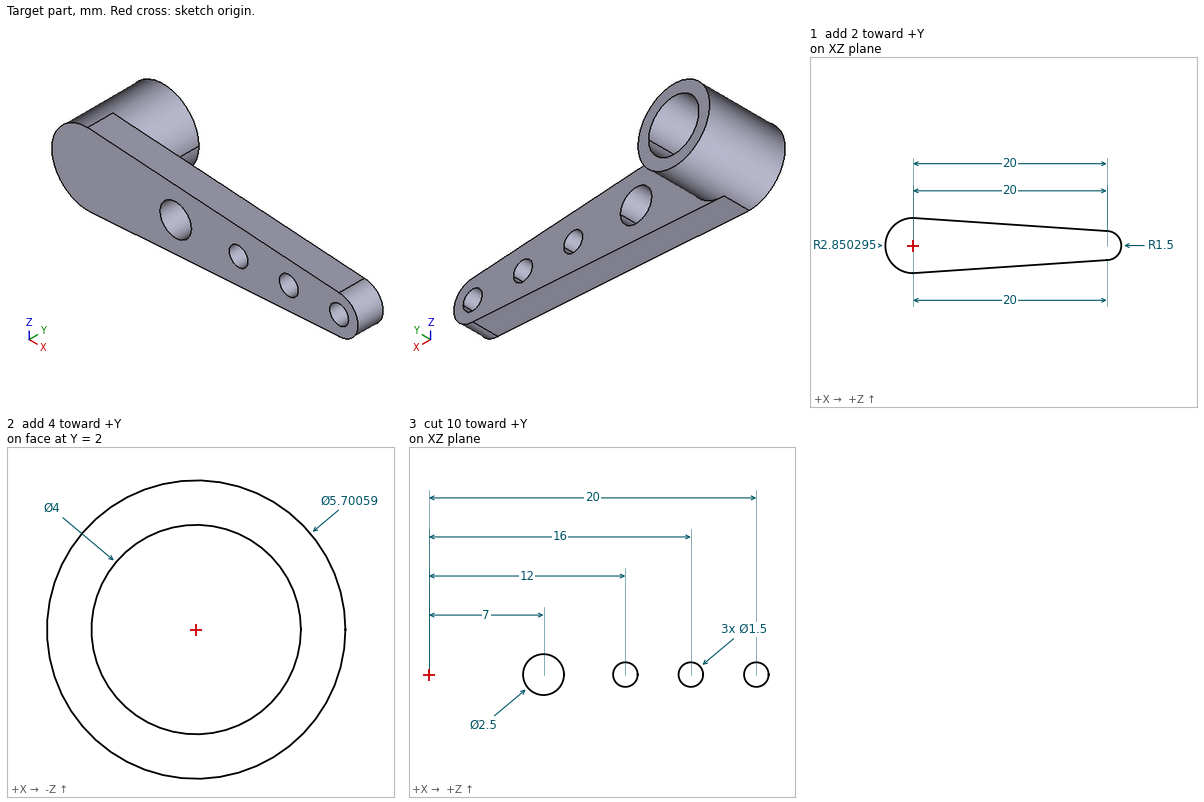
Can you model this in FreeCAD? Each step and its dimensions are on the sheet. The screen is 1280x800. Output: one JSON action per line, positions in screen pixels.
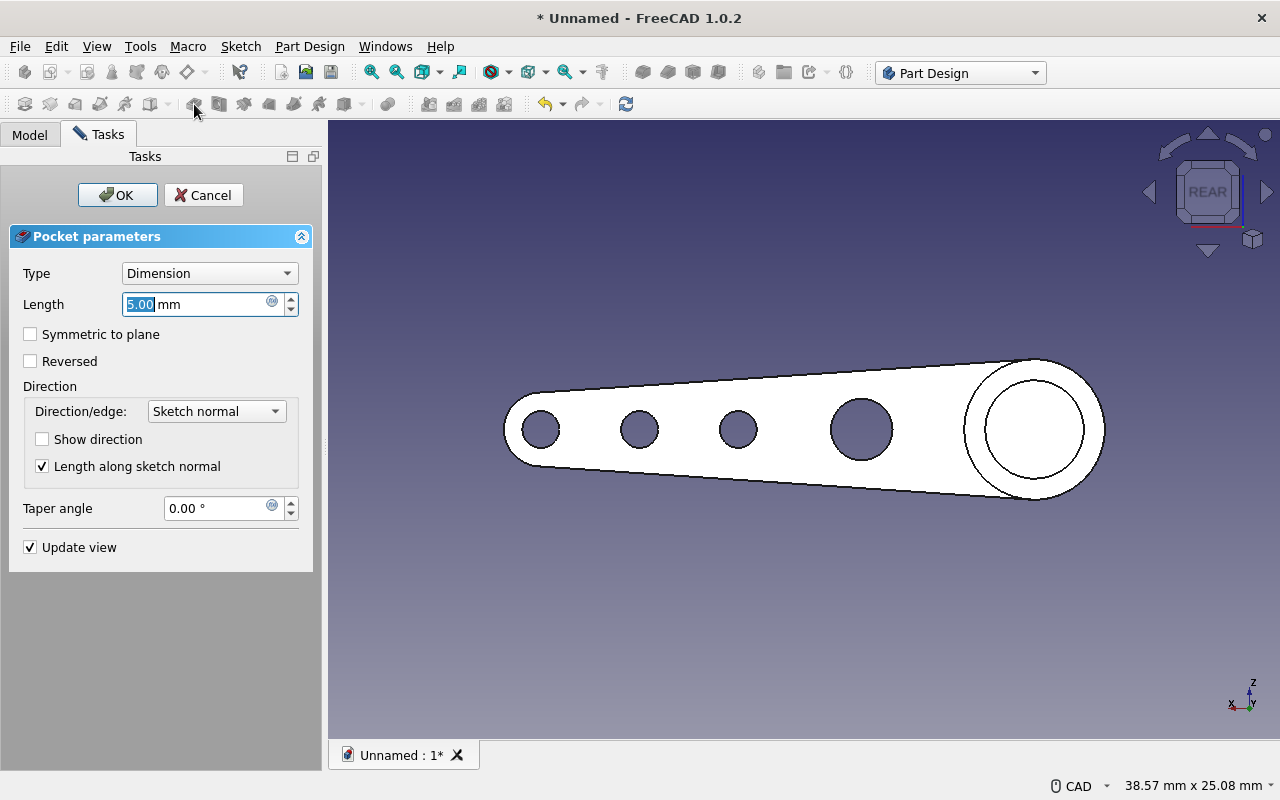
{"action": "type", "text": "10"}
{"action": "key", "text": "Tab"}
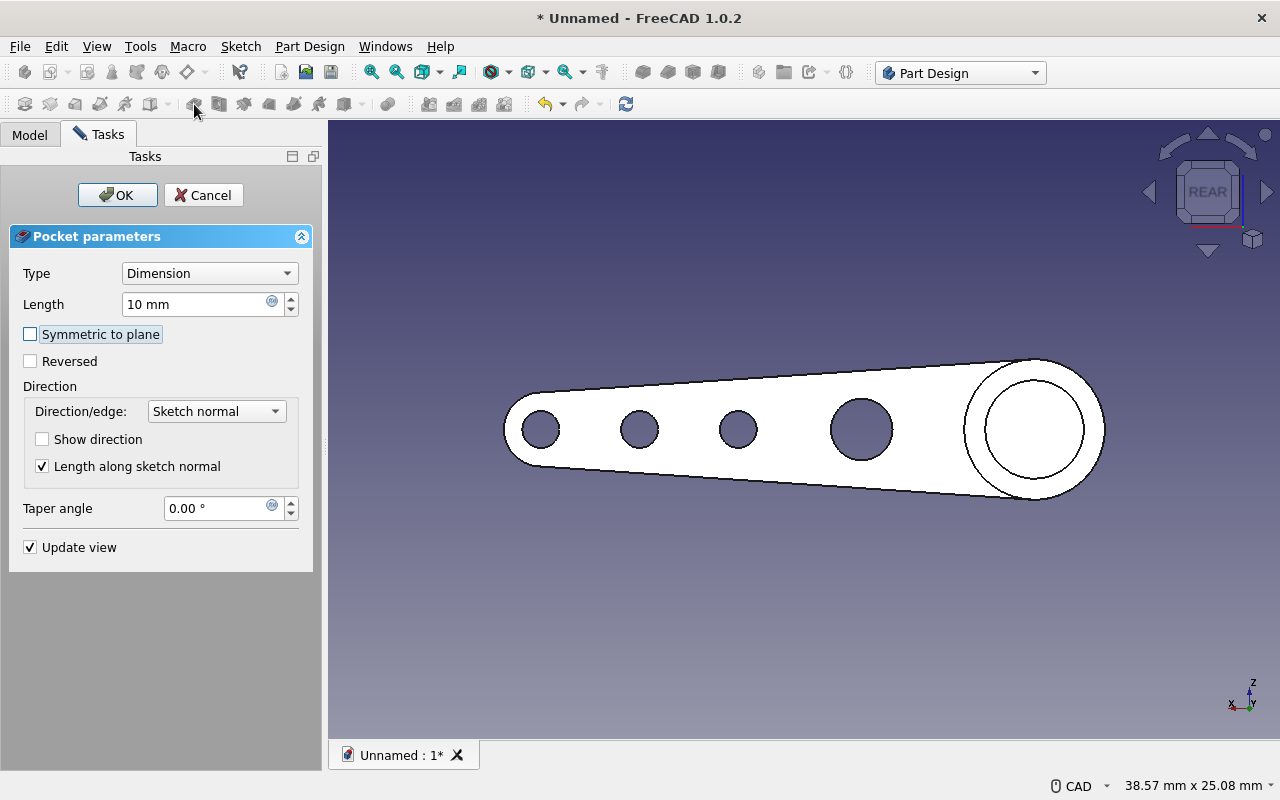
{"action": "left_click", "coordinate": [118, 195]}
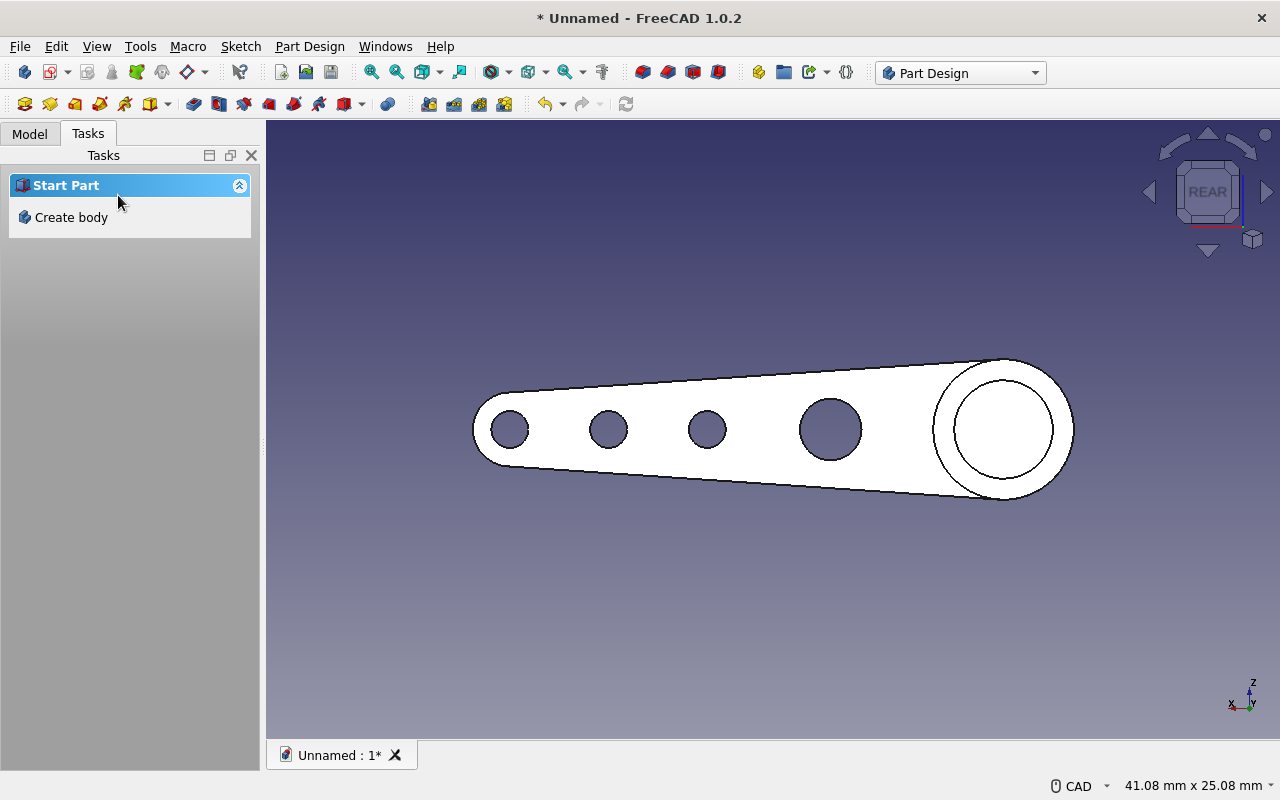
{"action": "key", "text": "0"}